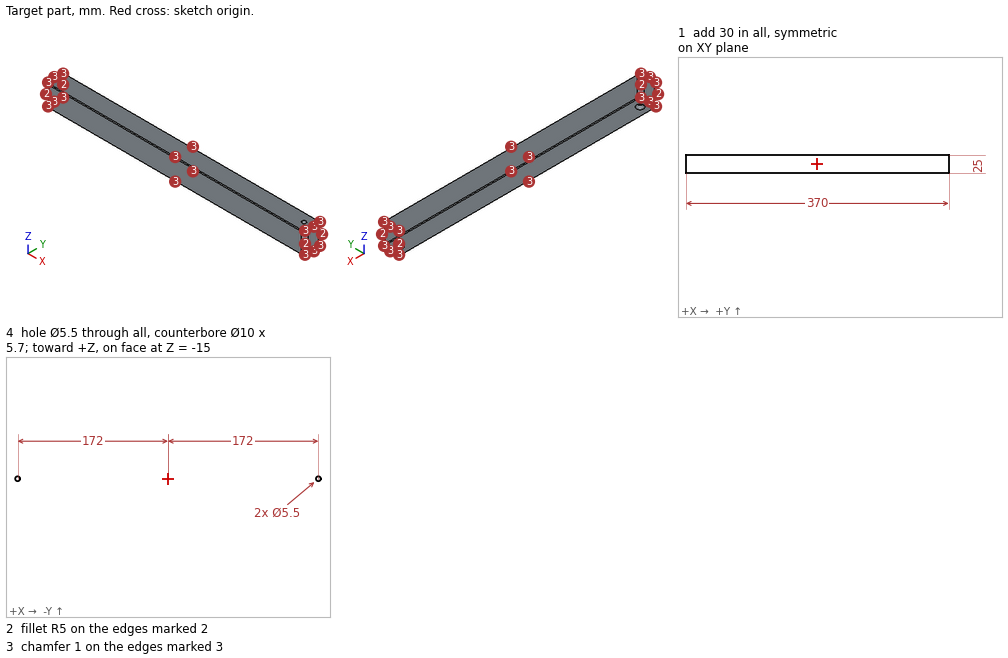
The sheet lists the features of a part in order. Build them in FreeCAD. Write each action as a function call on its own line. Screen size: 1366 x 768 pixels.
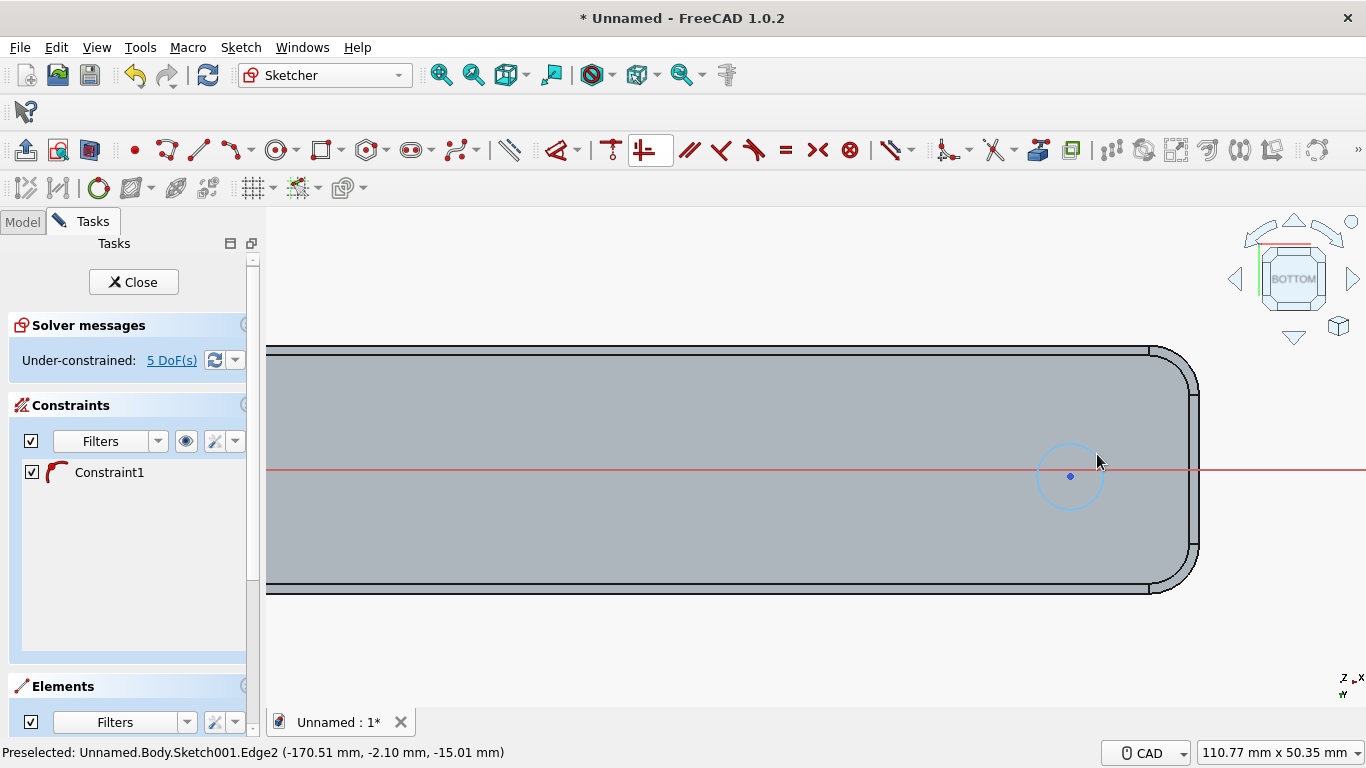
click(1093, 453)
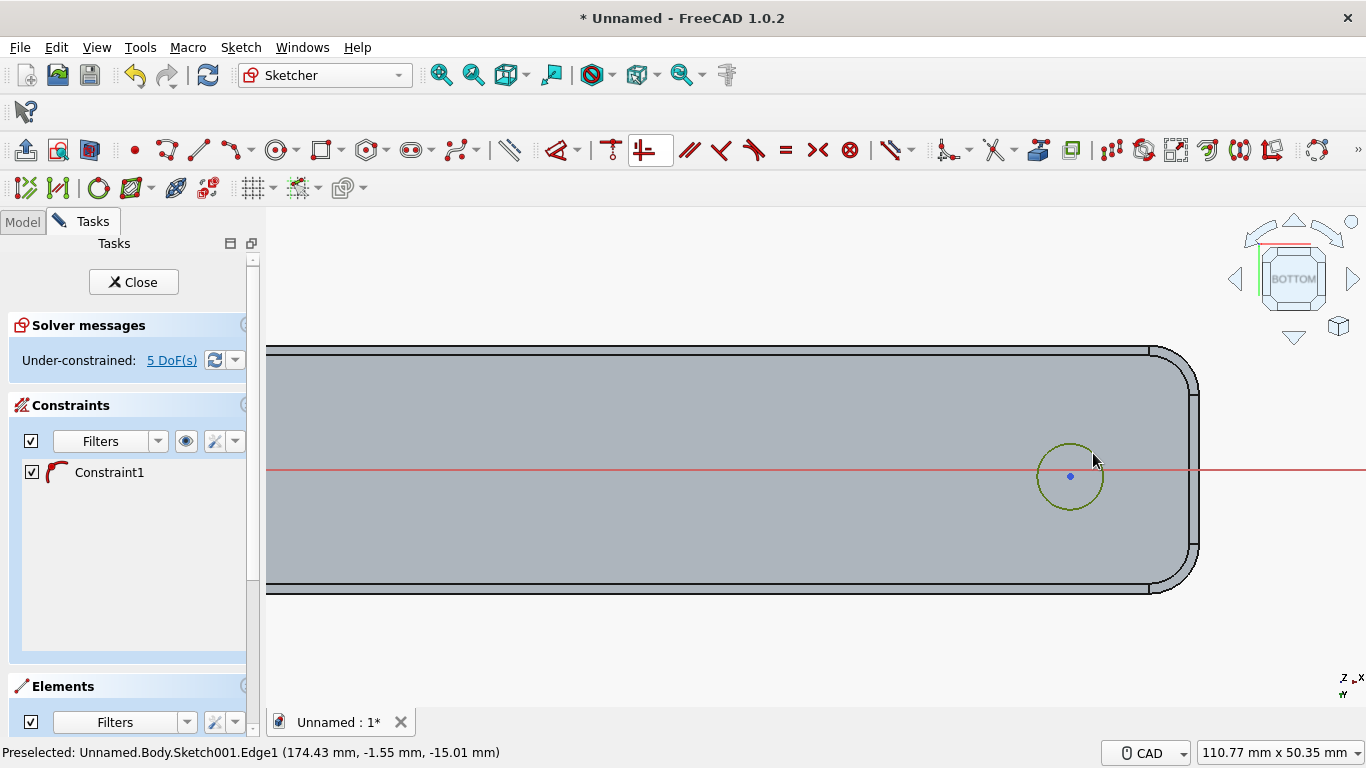
scroll(1098, 454, down, 8)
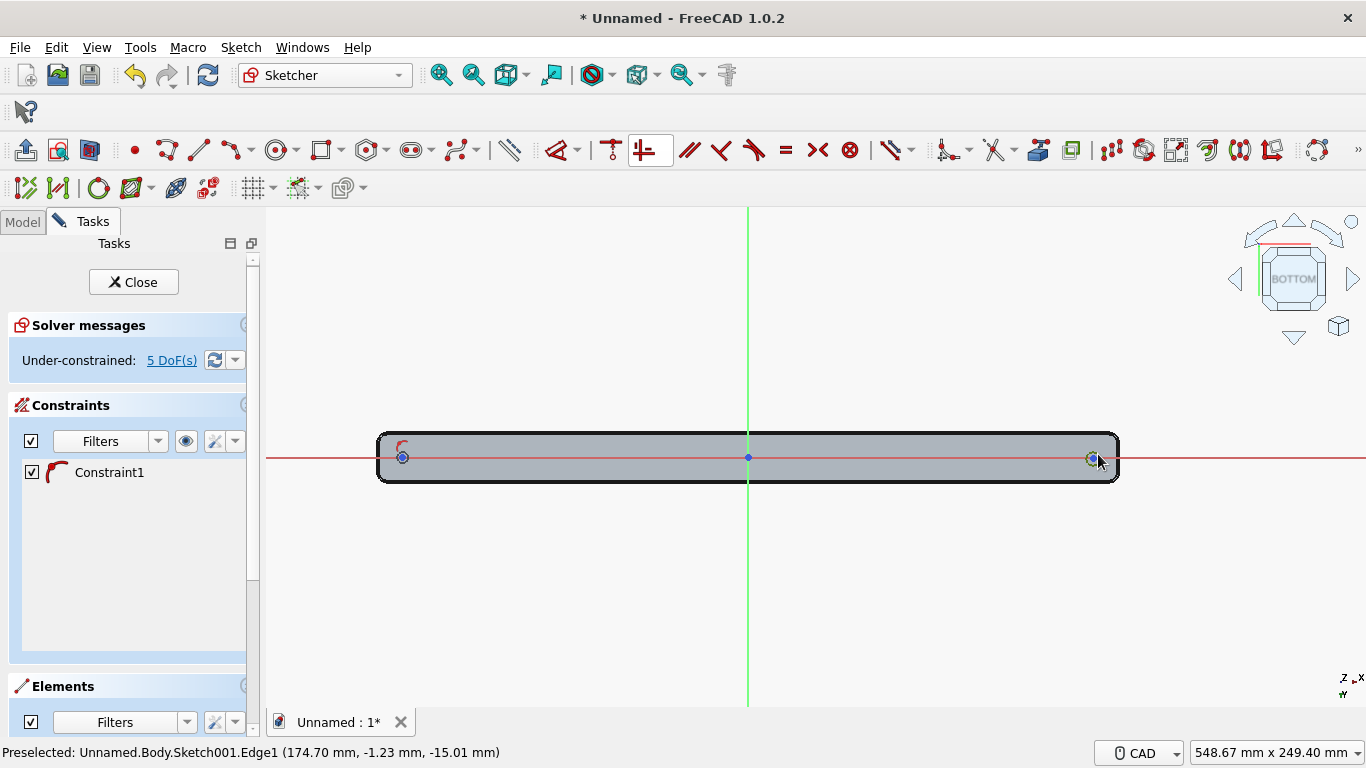
scroll(407, 454, up, 7)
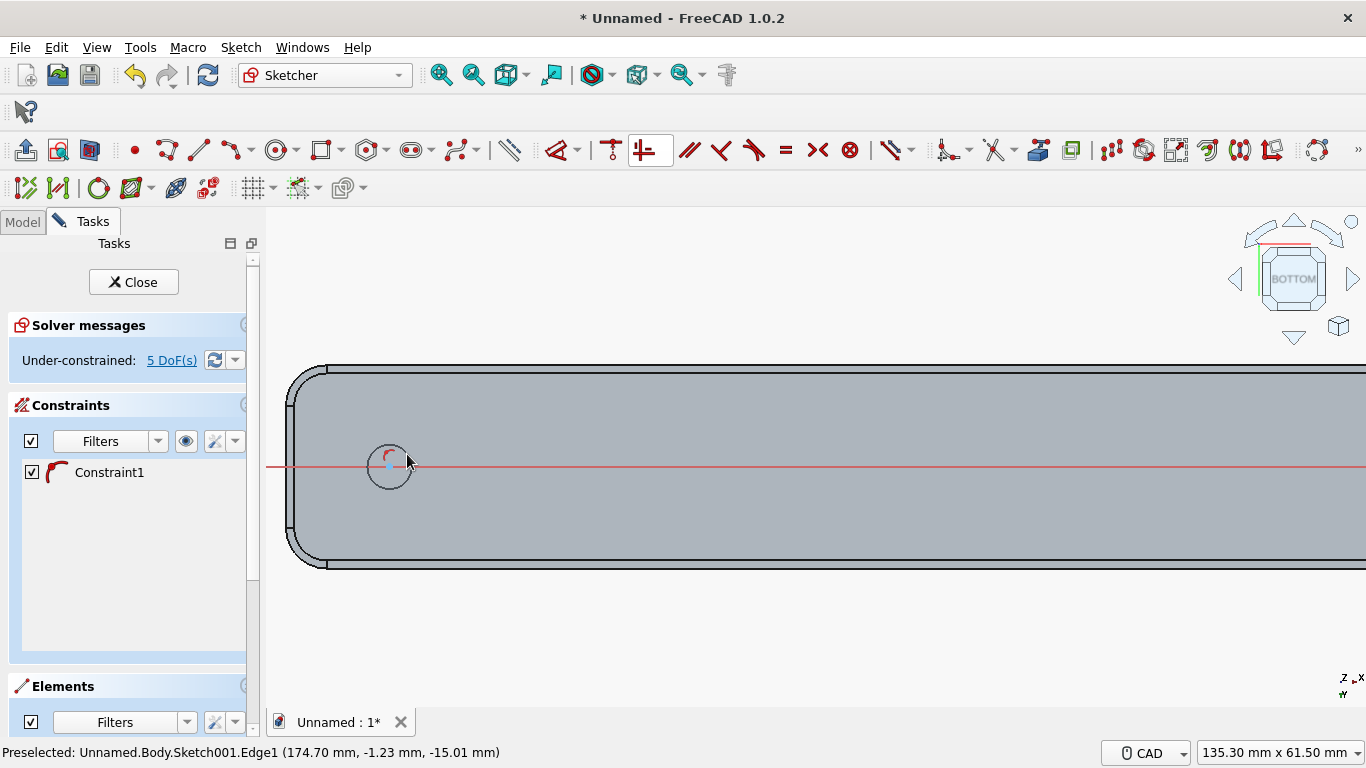
click(405, 451)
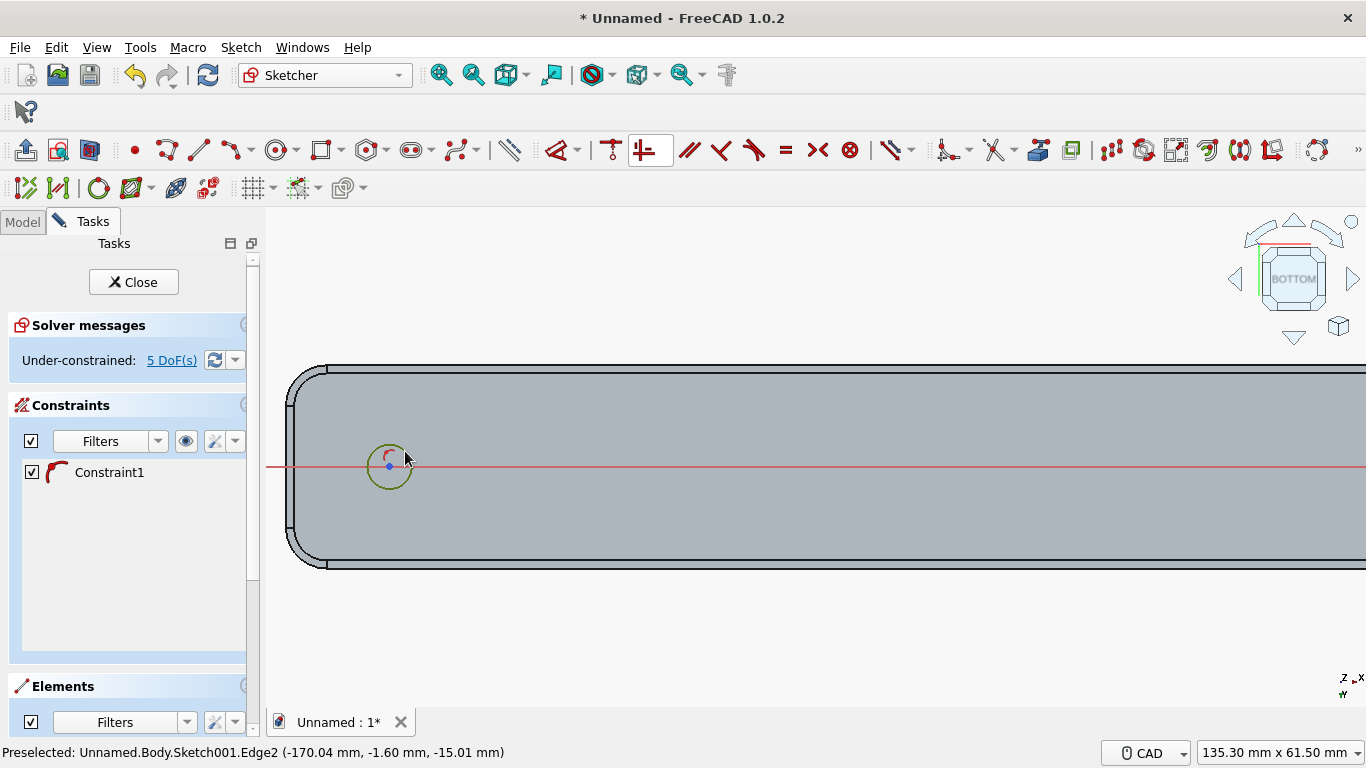
click(786, 150)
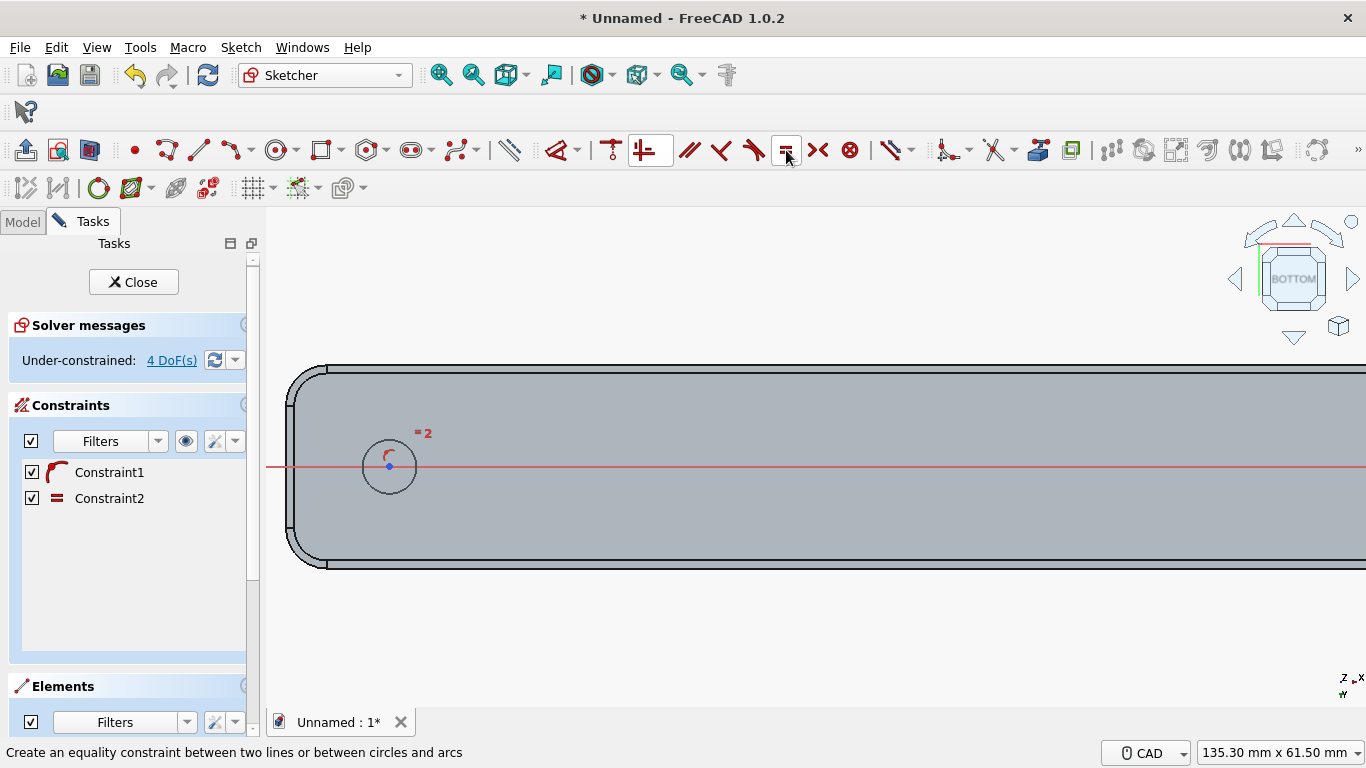
scroll(406, 454, down, 7)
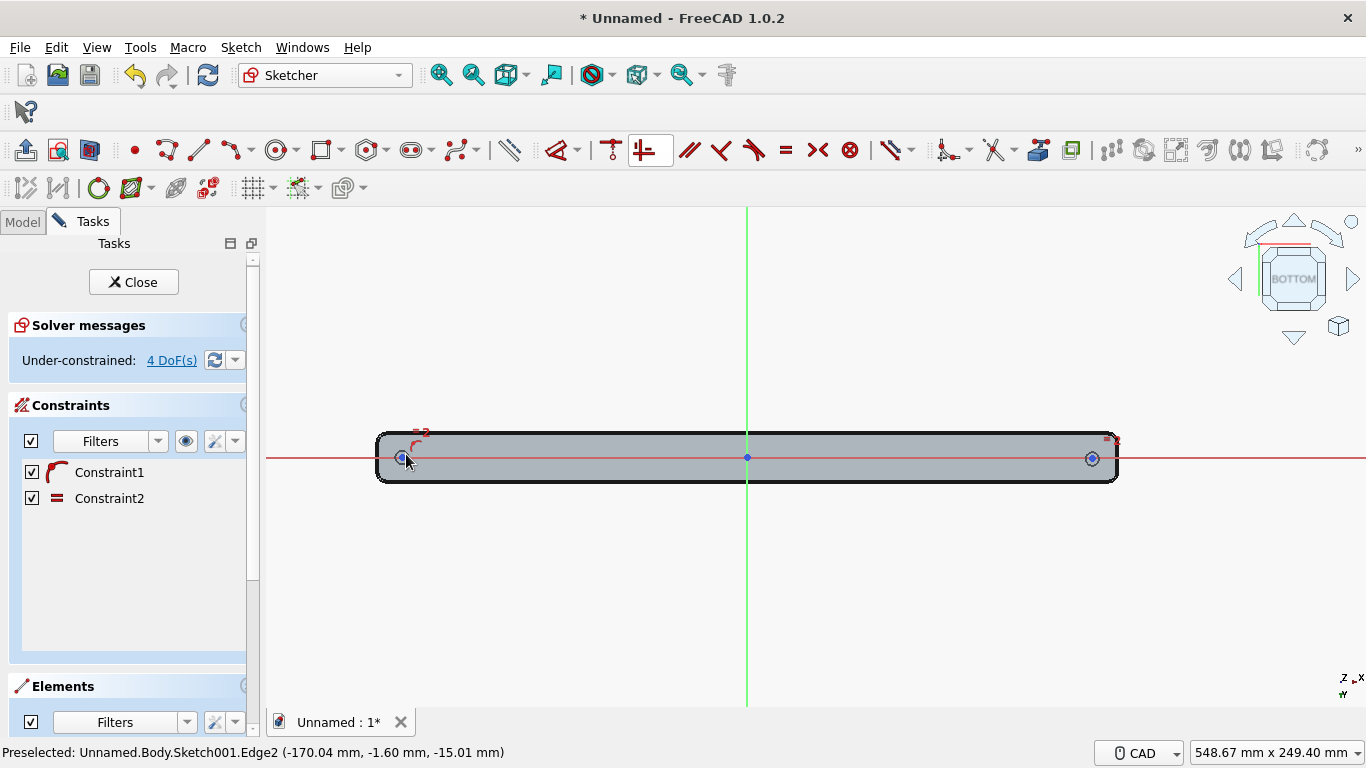
click(1092, 459)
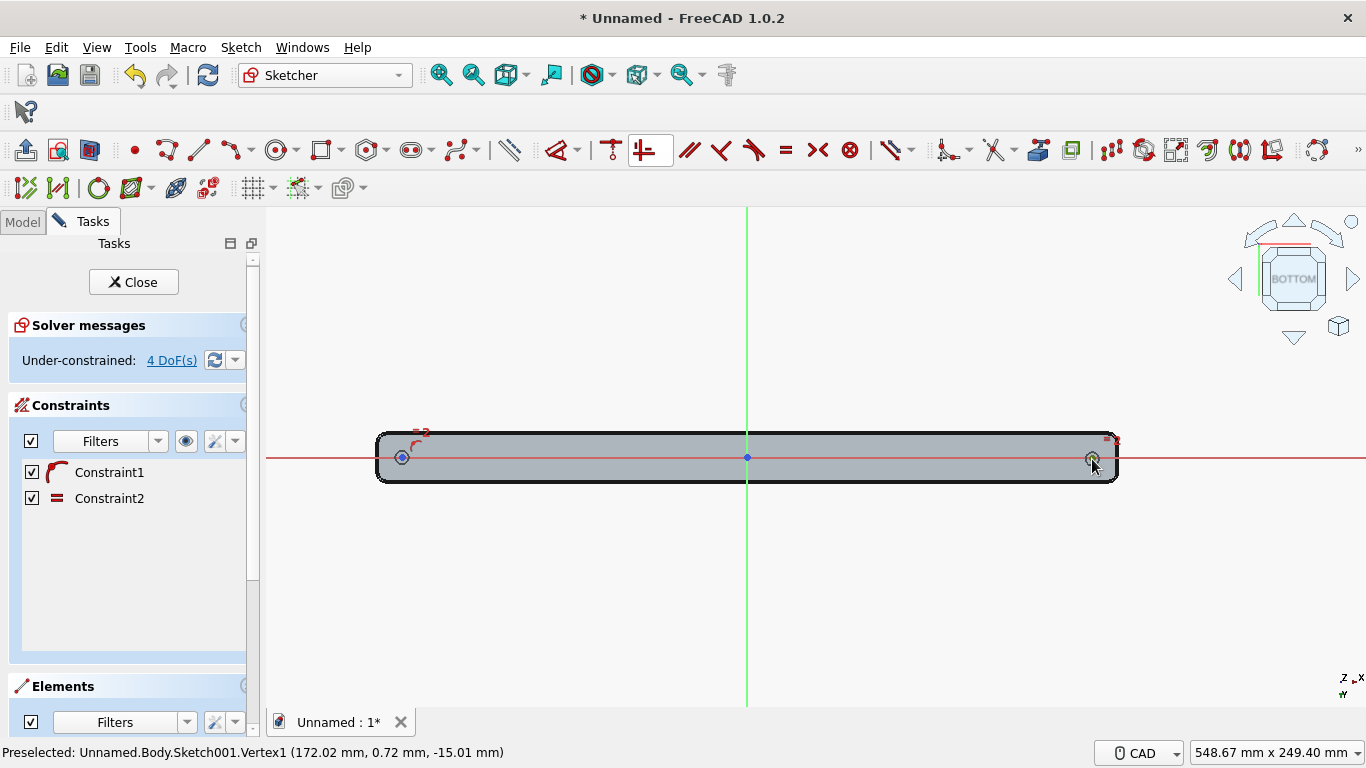
click(359, 458)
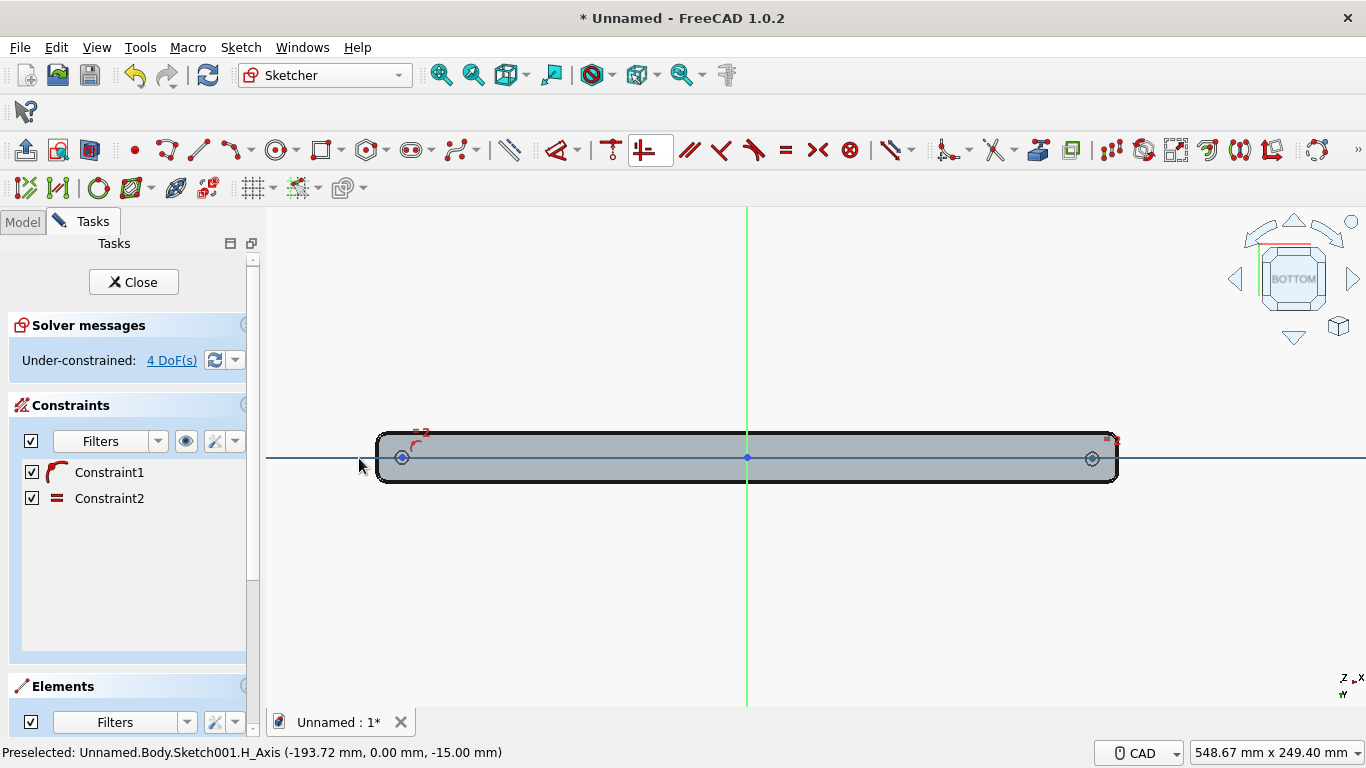
click(612, 150)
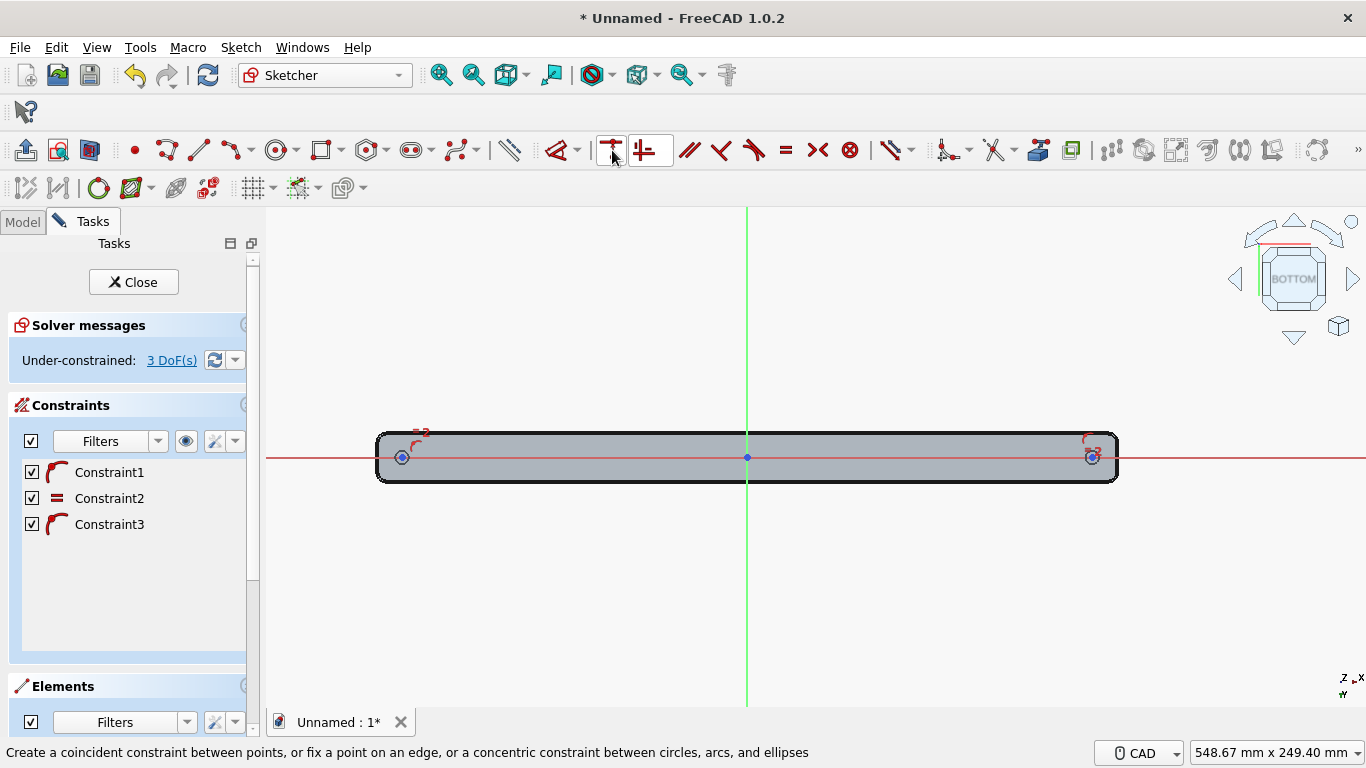
click(556, 150)